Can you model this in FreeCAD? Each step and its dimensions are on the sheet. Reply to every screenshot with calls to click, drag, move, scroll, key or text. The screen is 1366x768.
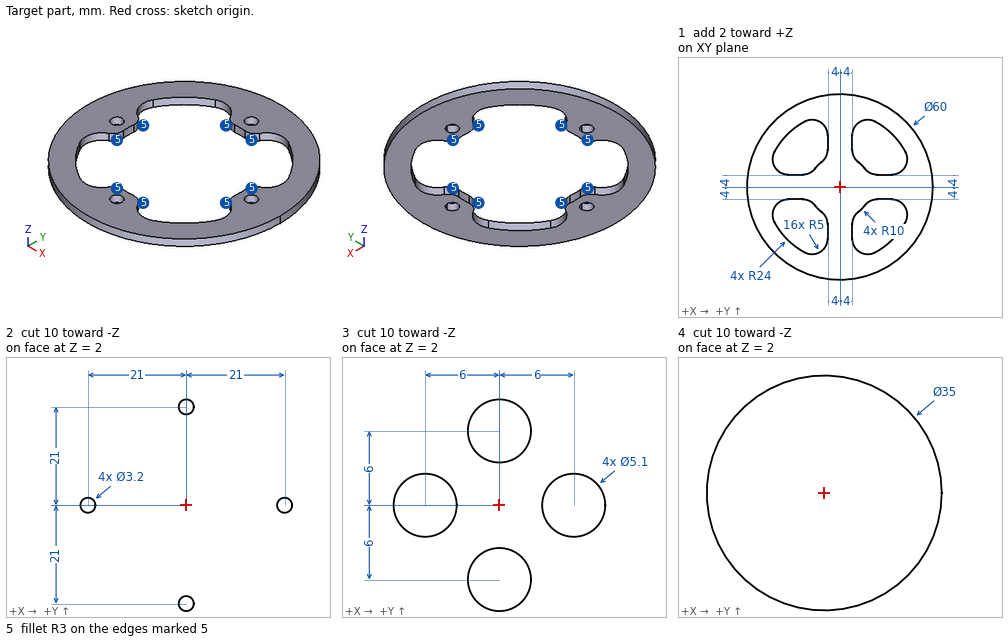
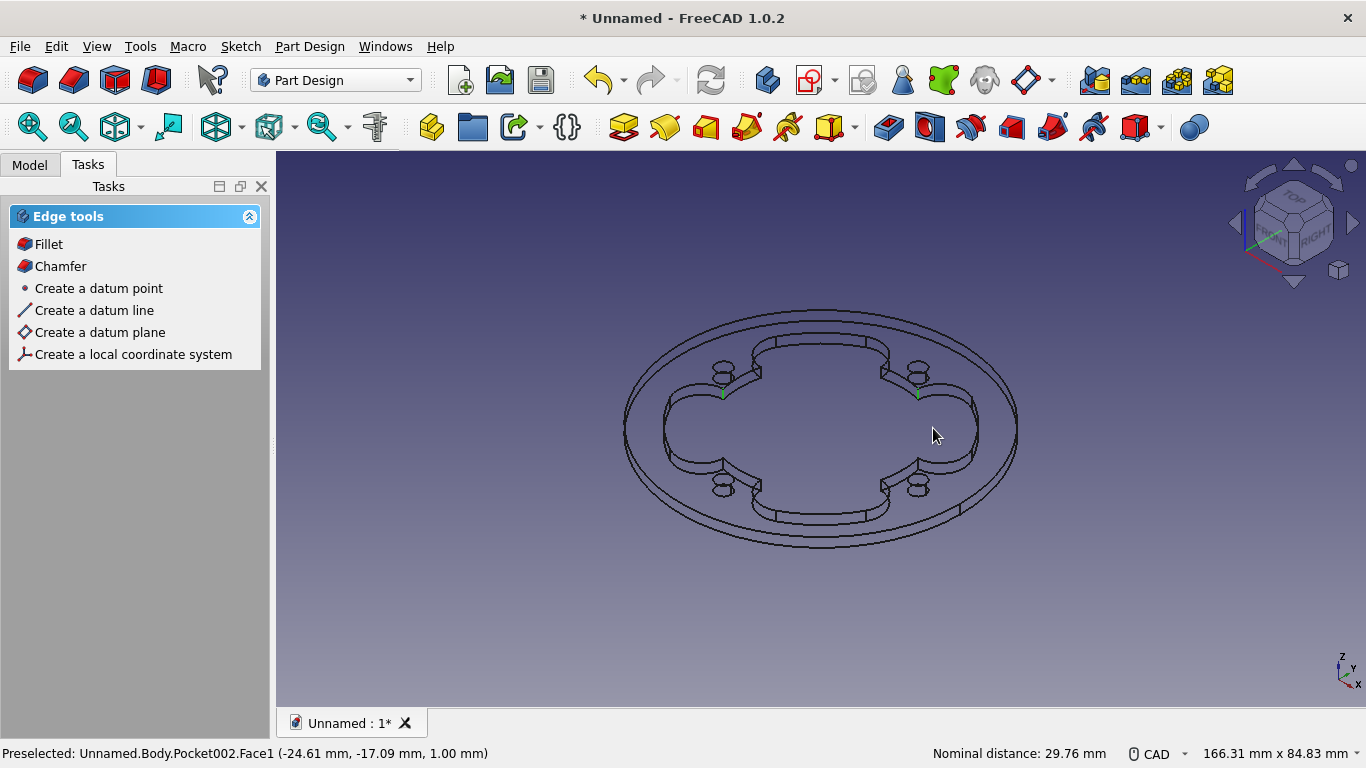
click(761, 487, ctrl)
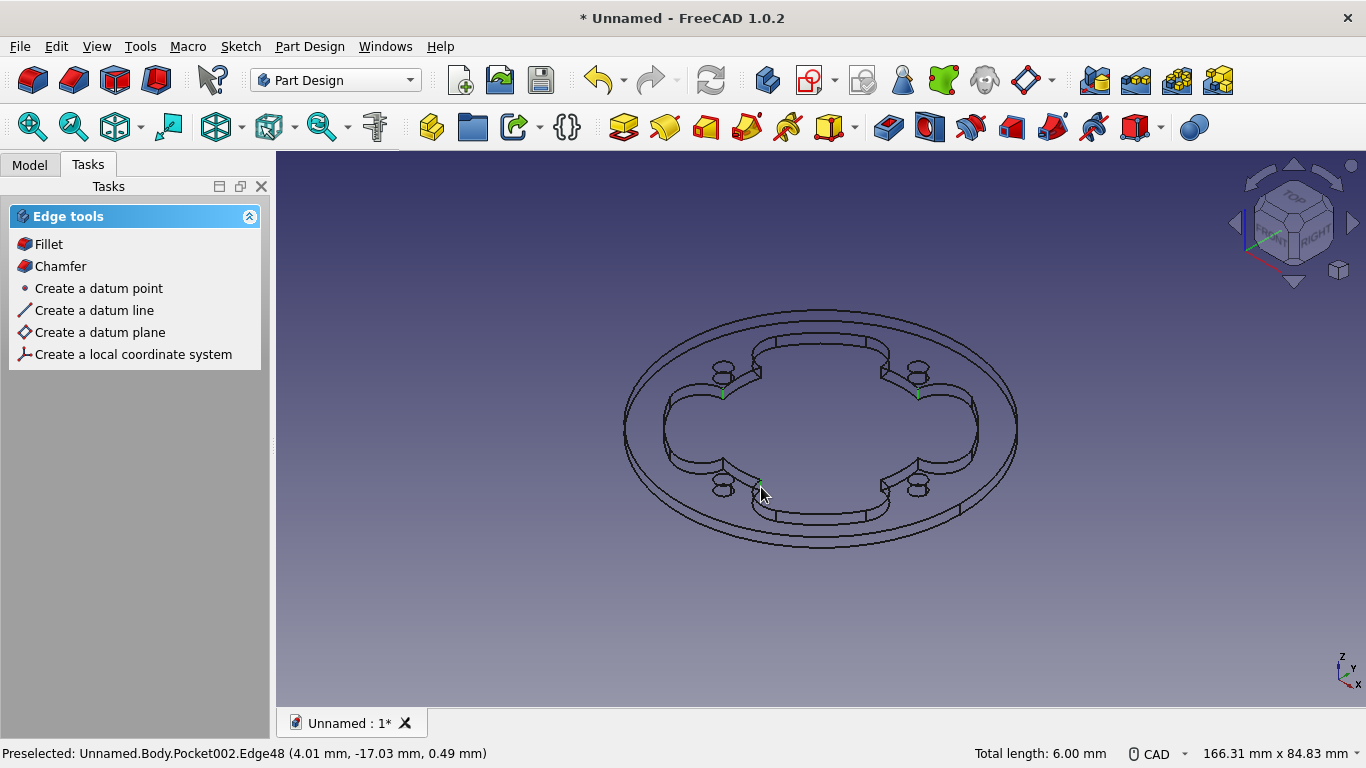
click(761, 373, ctrl)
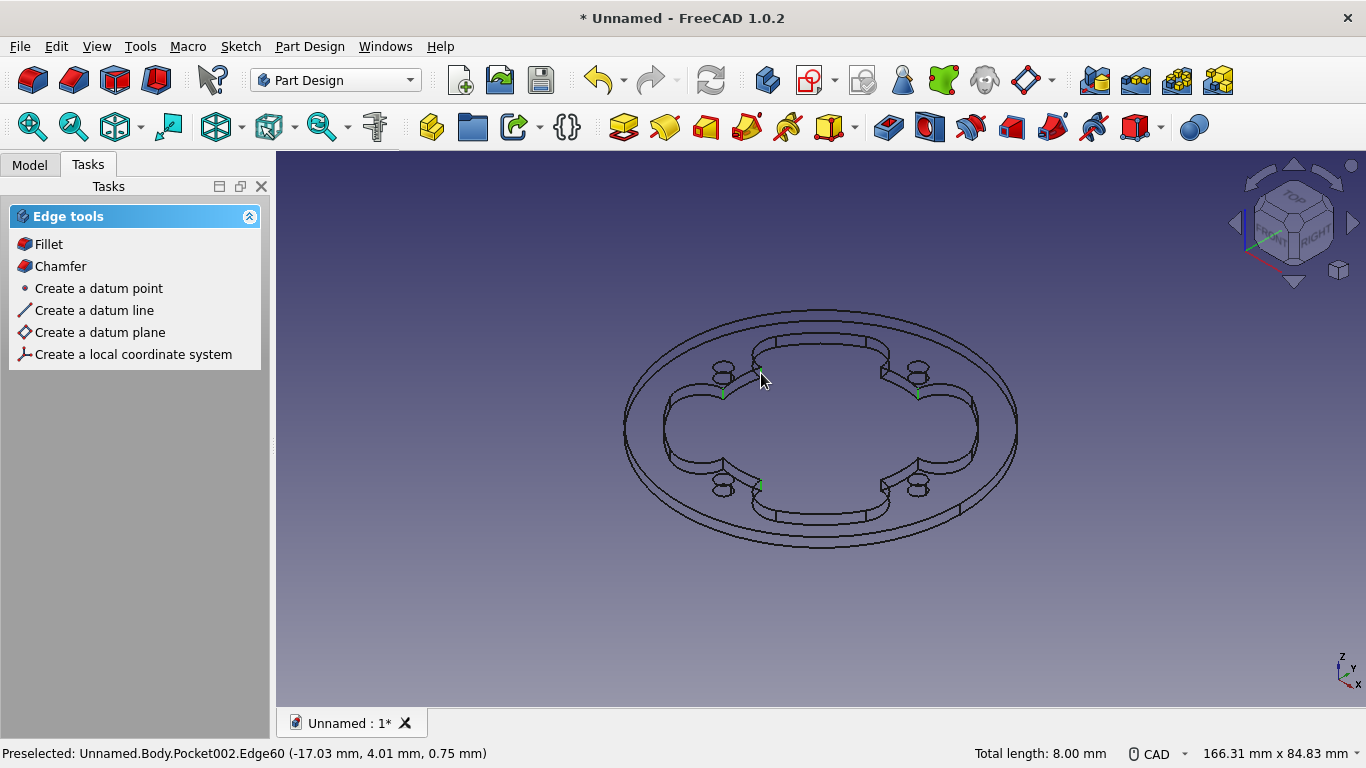
click(881, 373, ctrl)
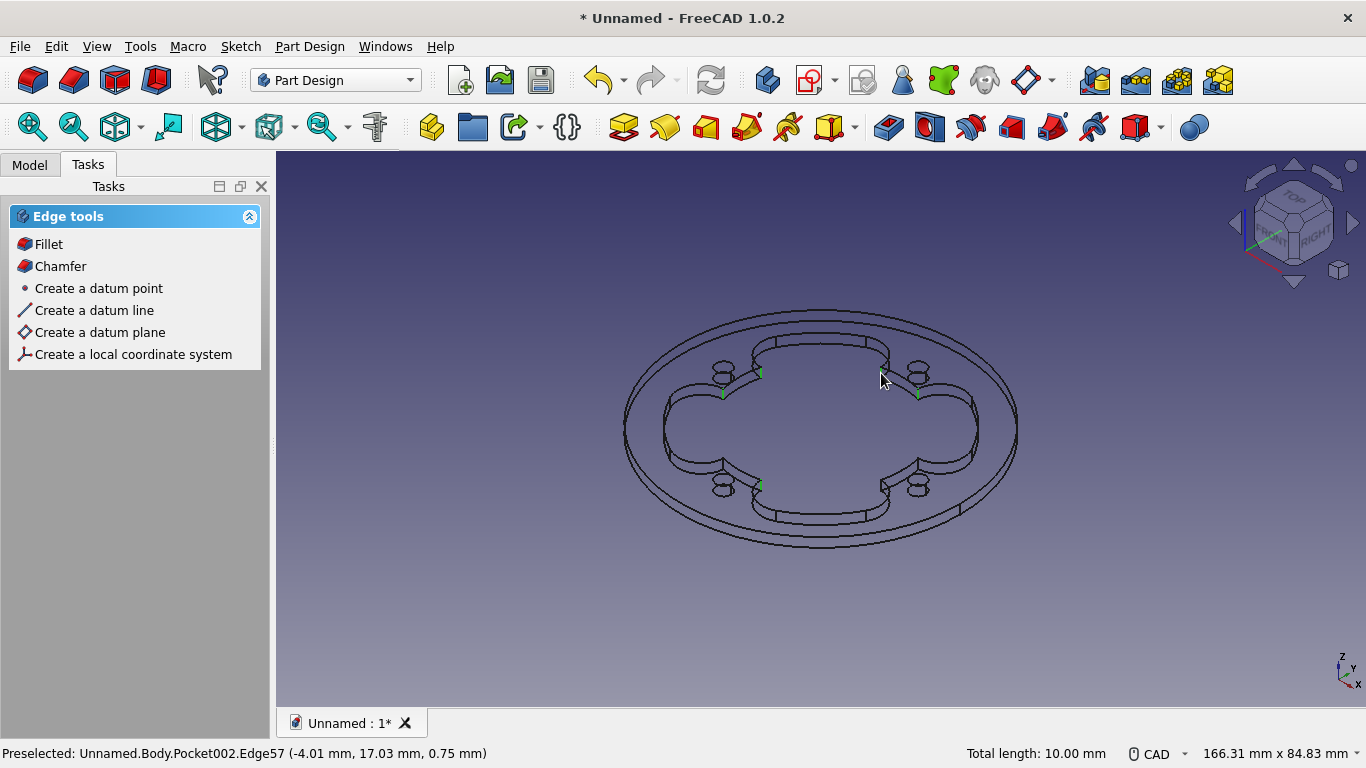
scroll(723, 463, up, 6)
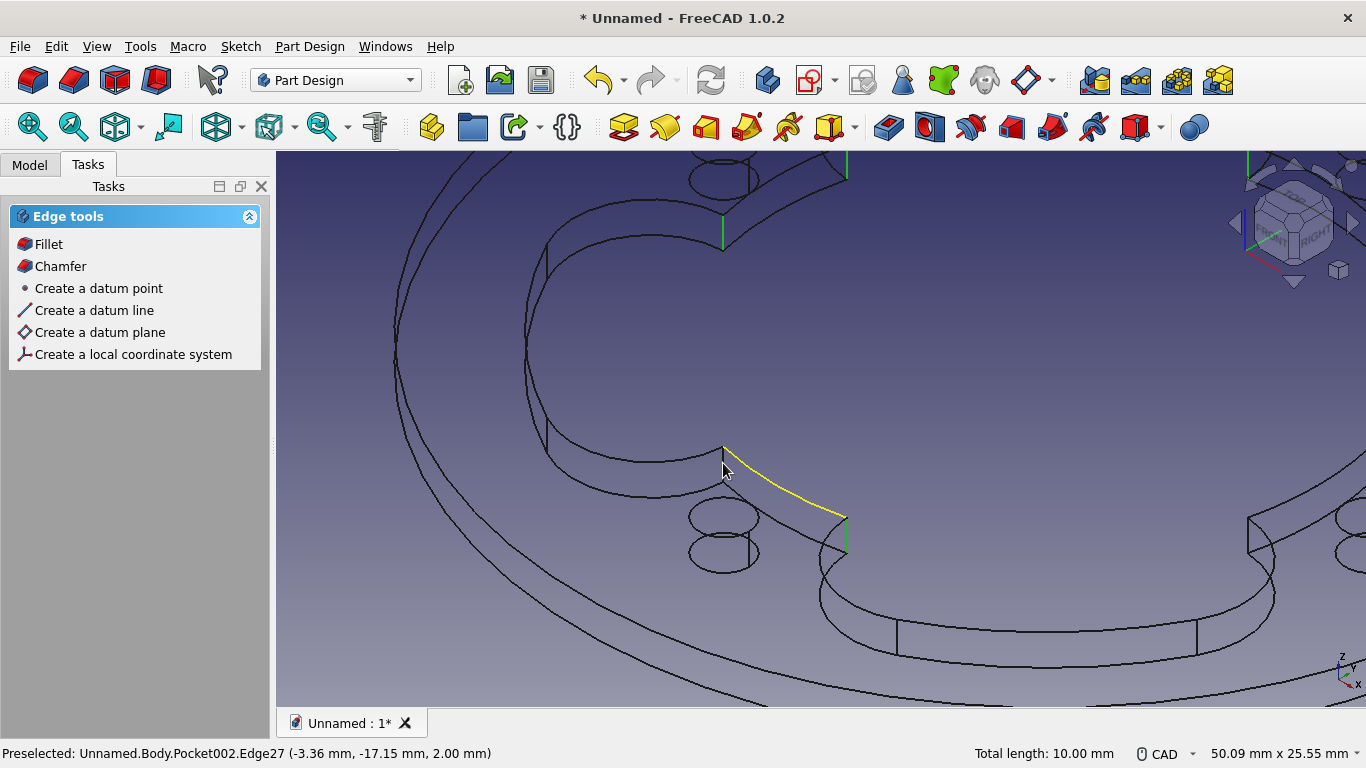
click(723, 463, ctrl)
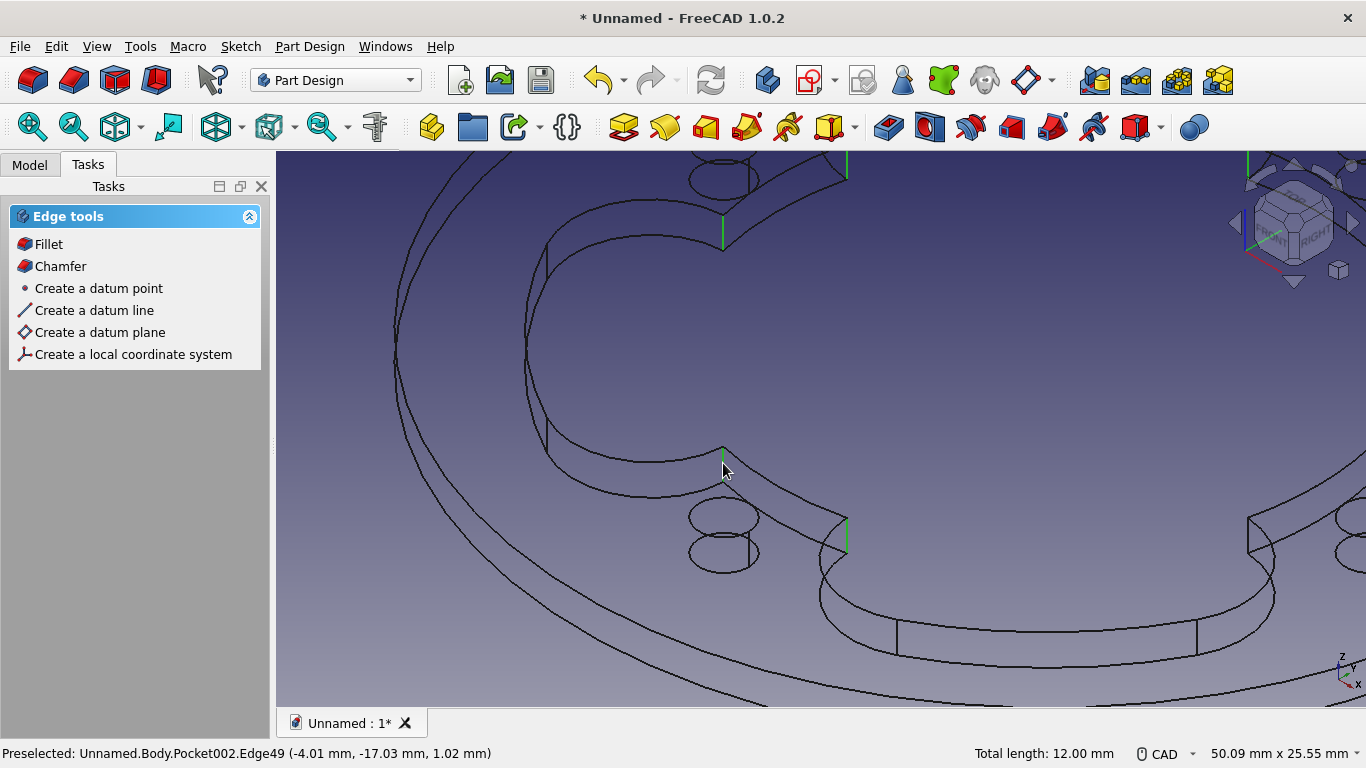
click(1248, 535, ctrl)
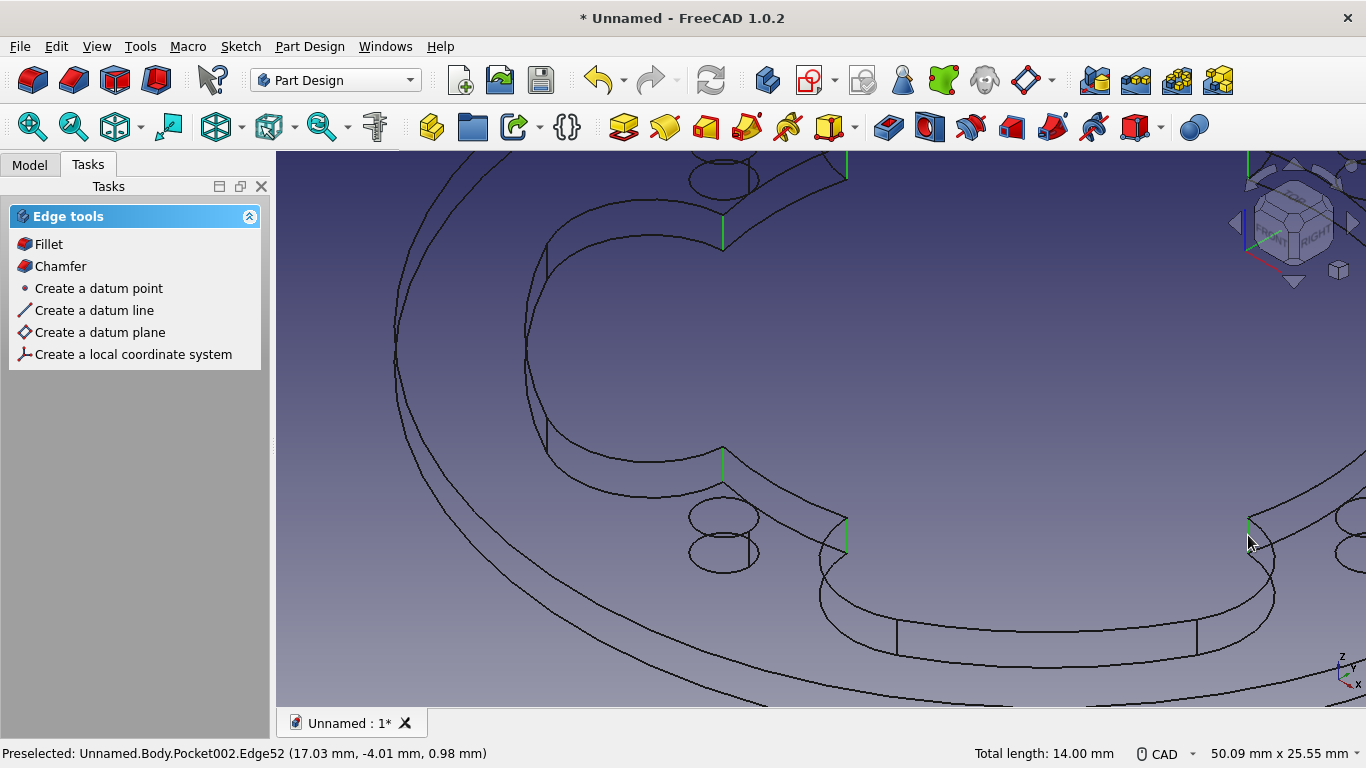
click(33, 128)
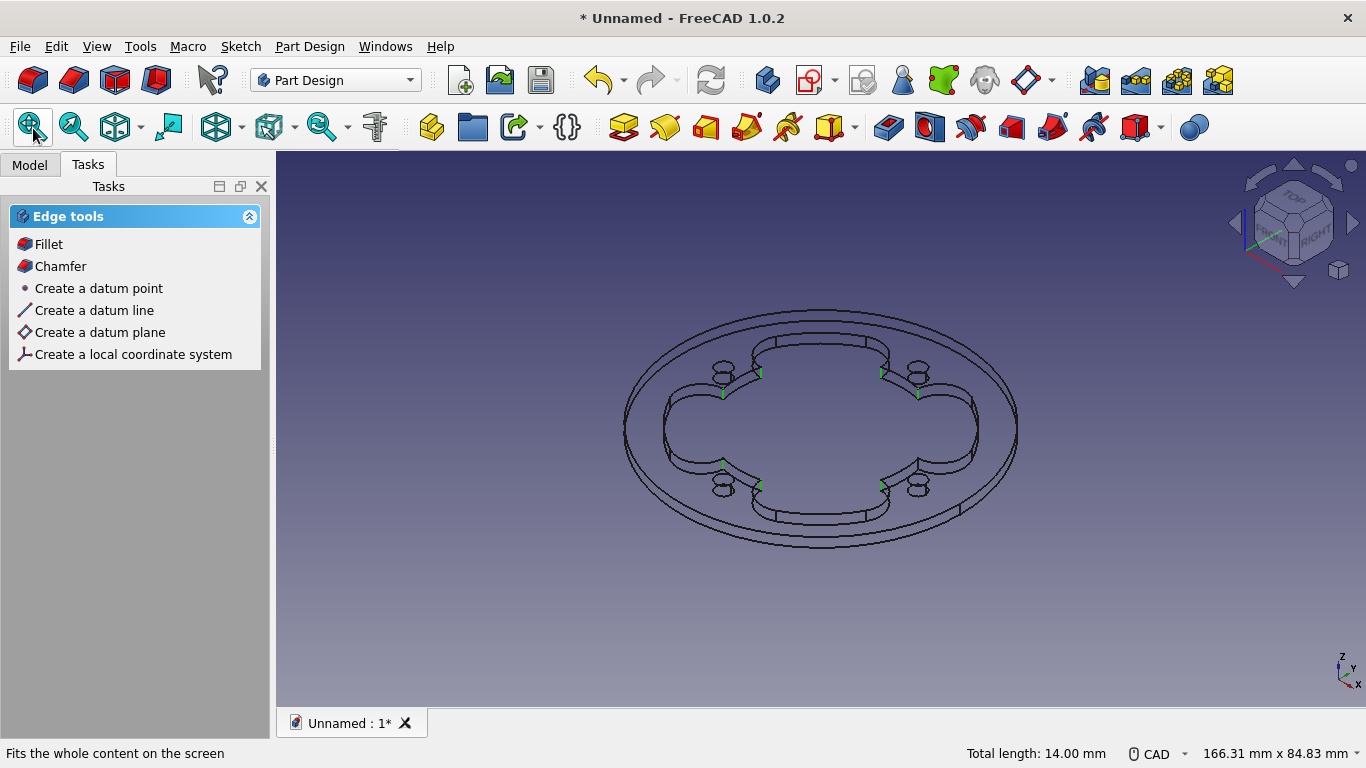
key(2)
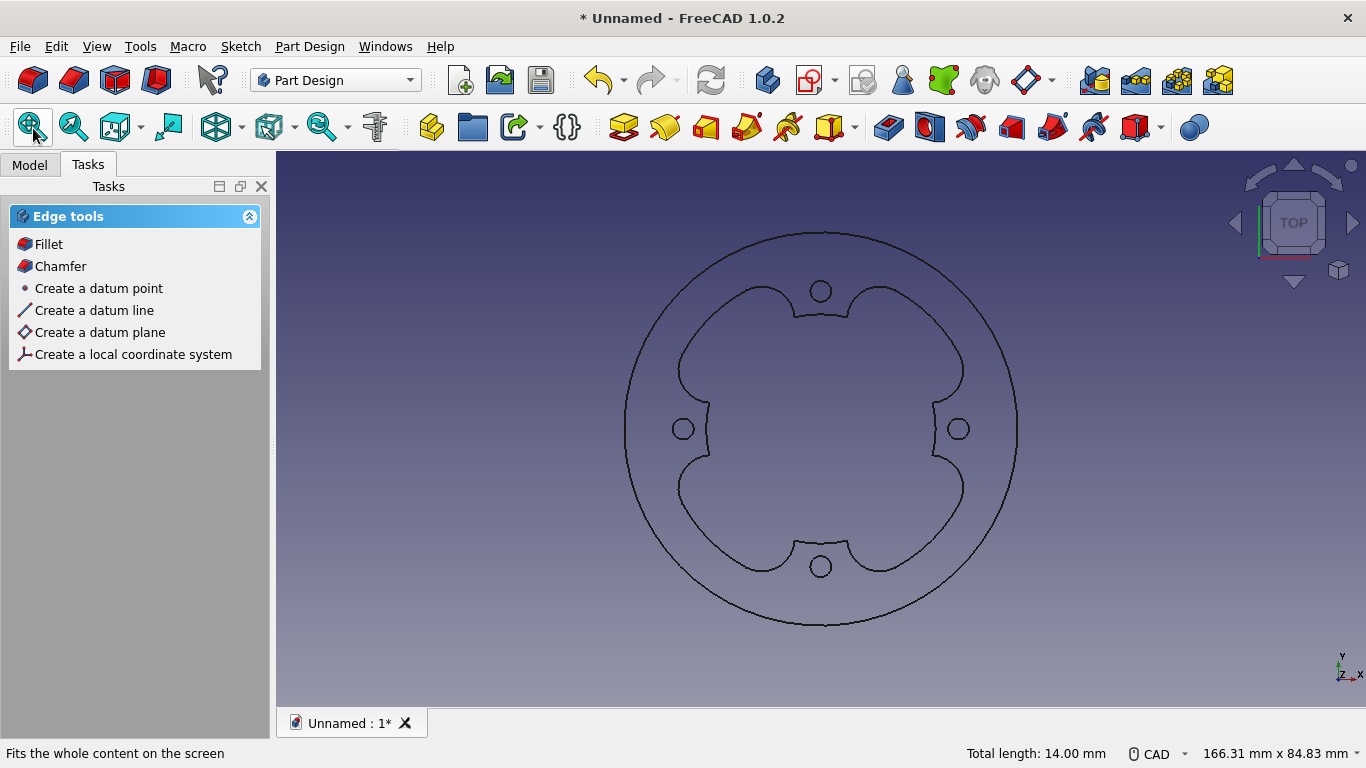
scroll(933, 402, up, 6)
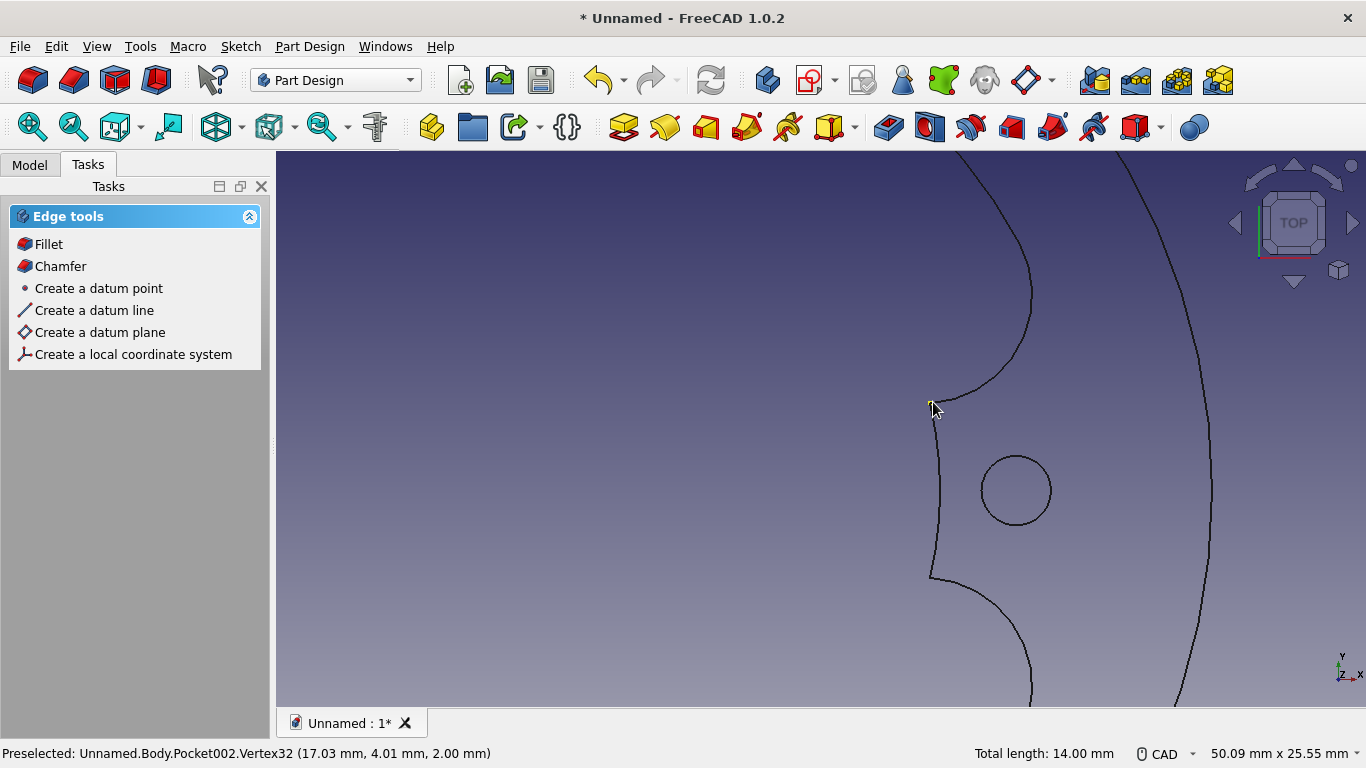
key(v)
key(f)